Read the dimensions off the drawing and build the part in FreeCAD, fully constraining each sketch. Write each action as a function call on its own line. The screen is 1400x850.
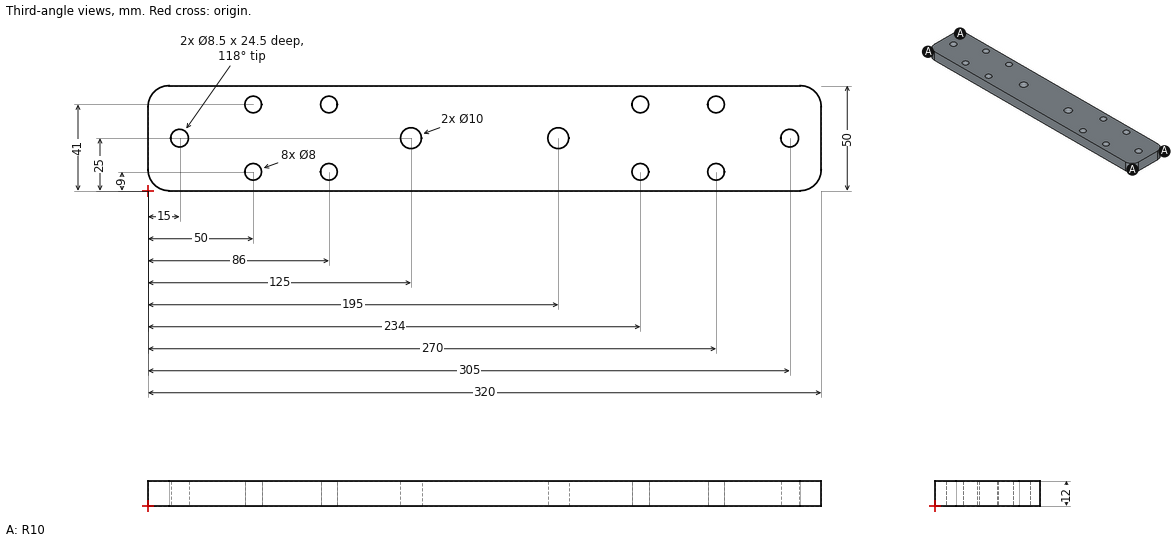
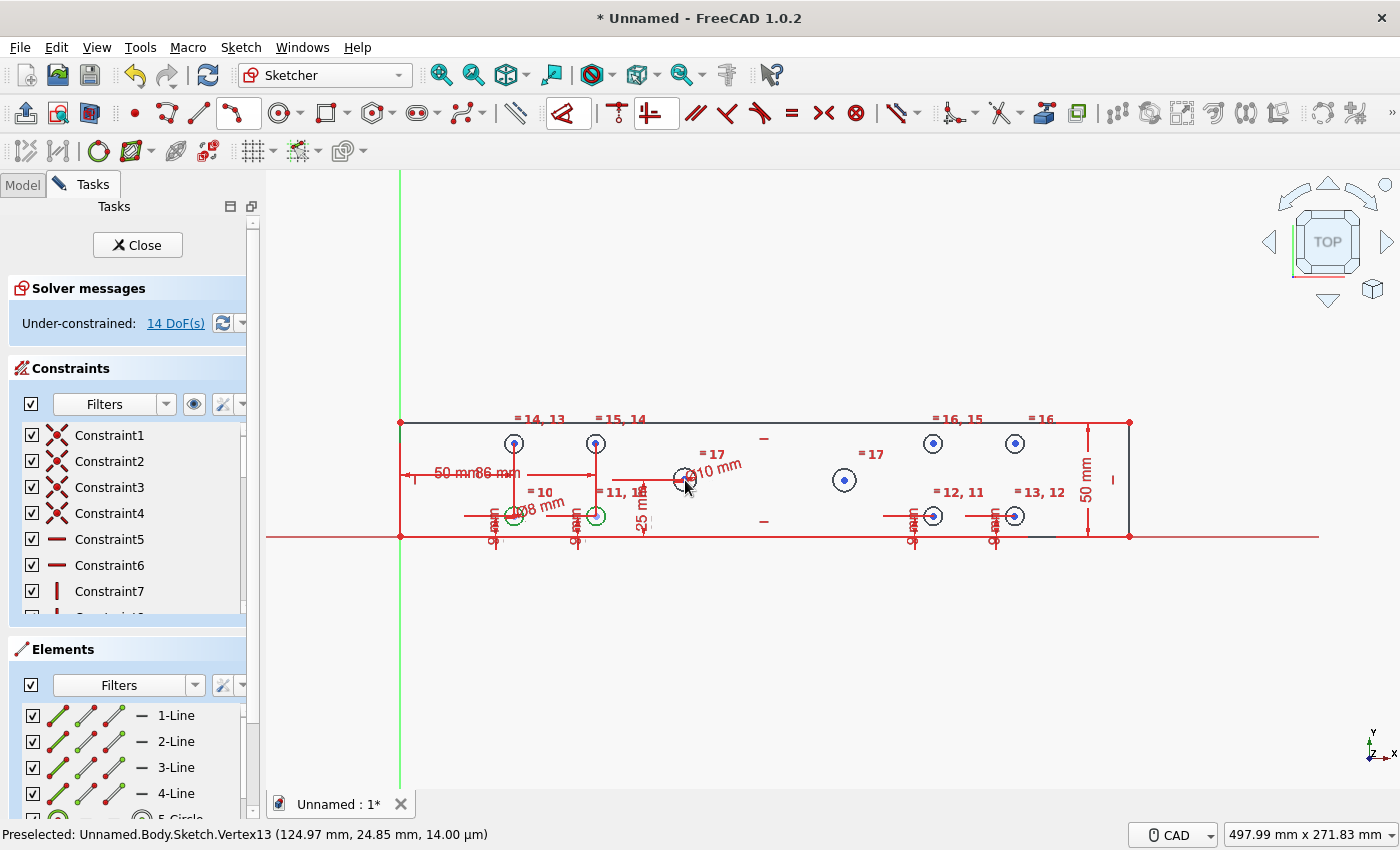
click(514, 444)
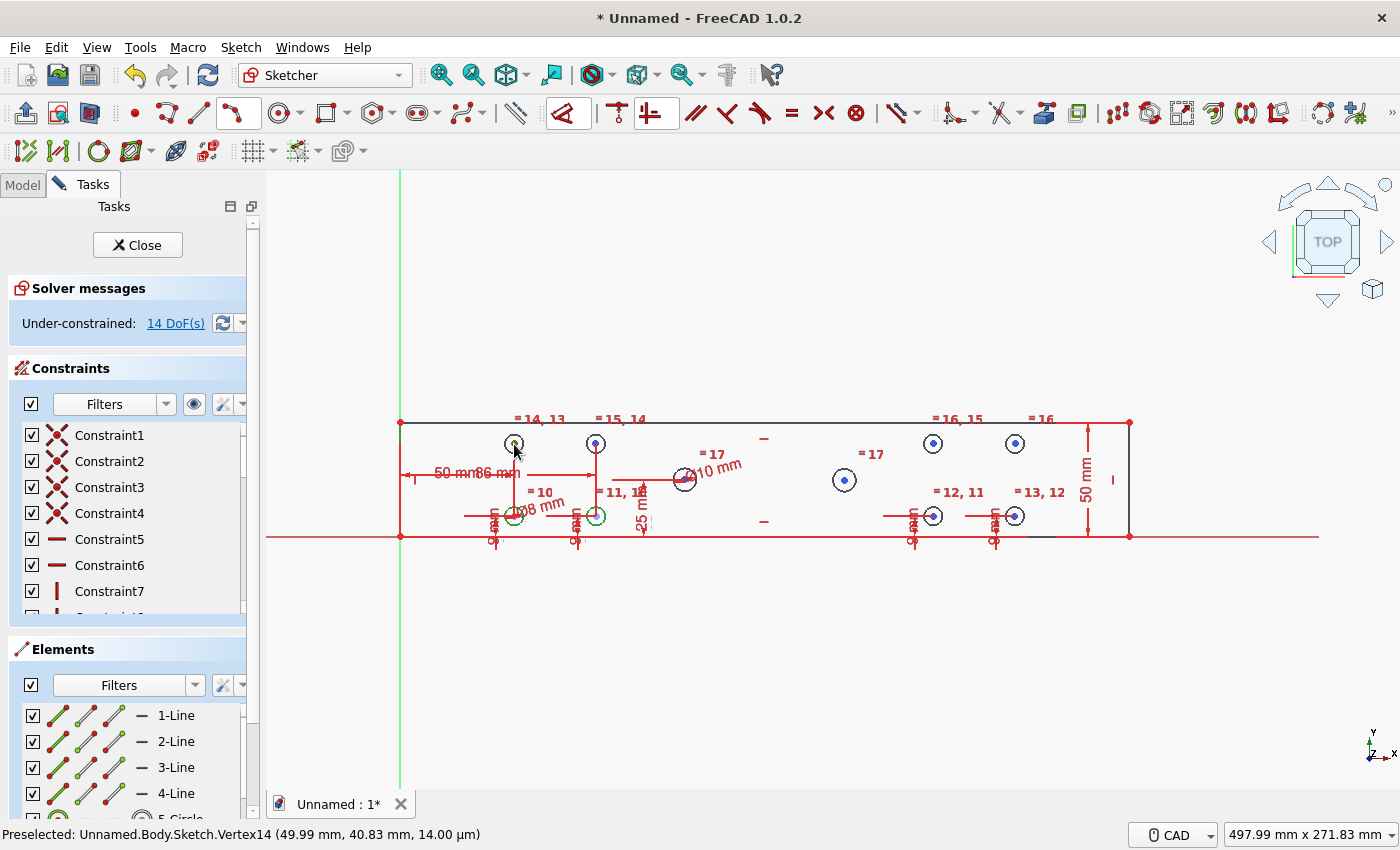
click(586, 114)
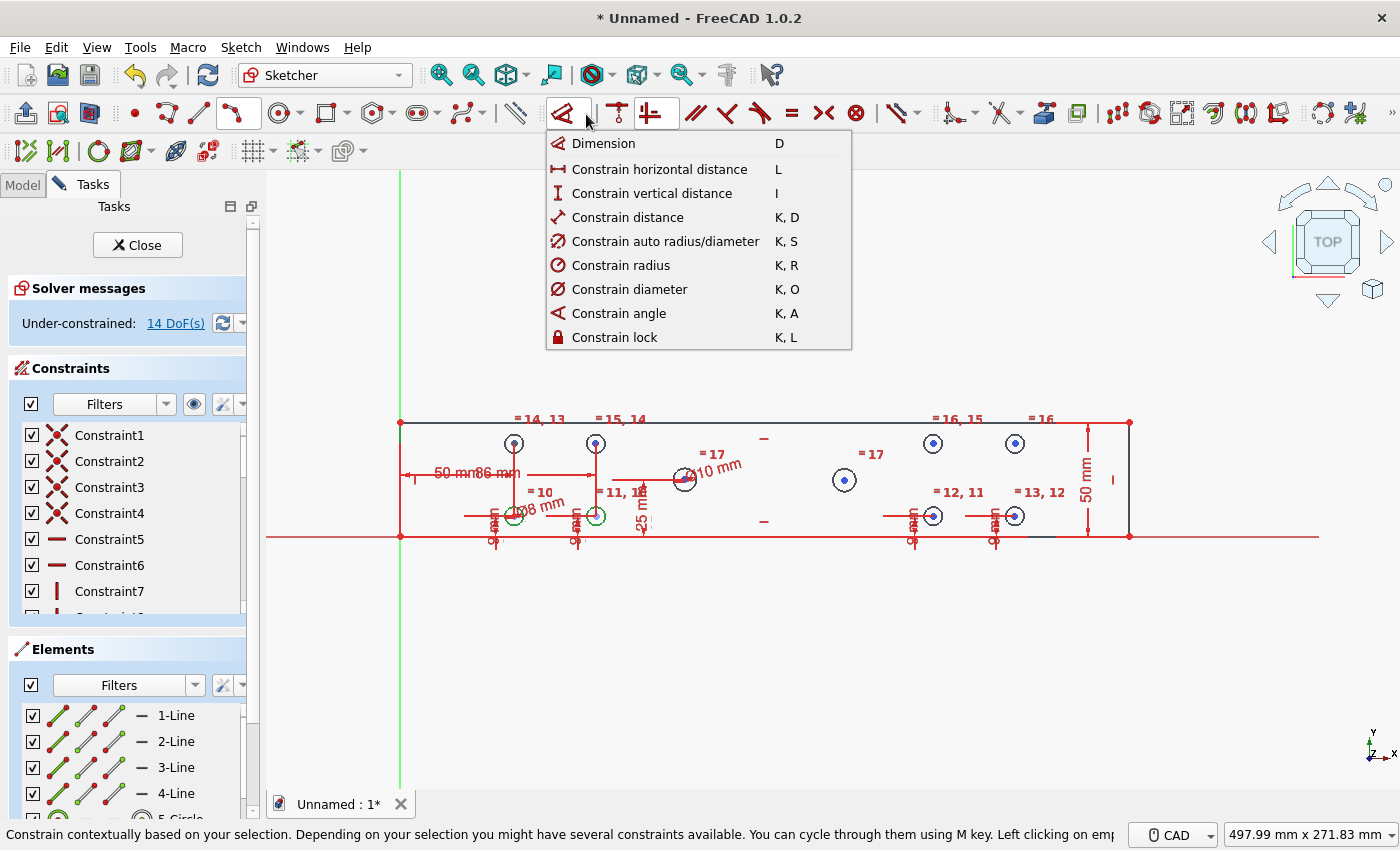
click(699, 169)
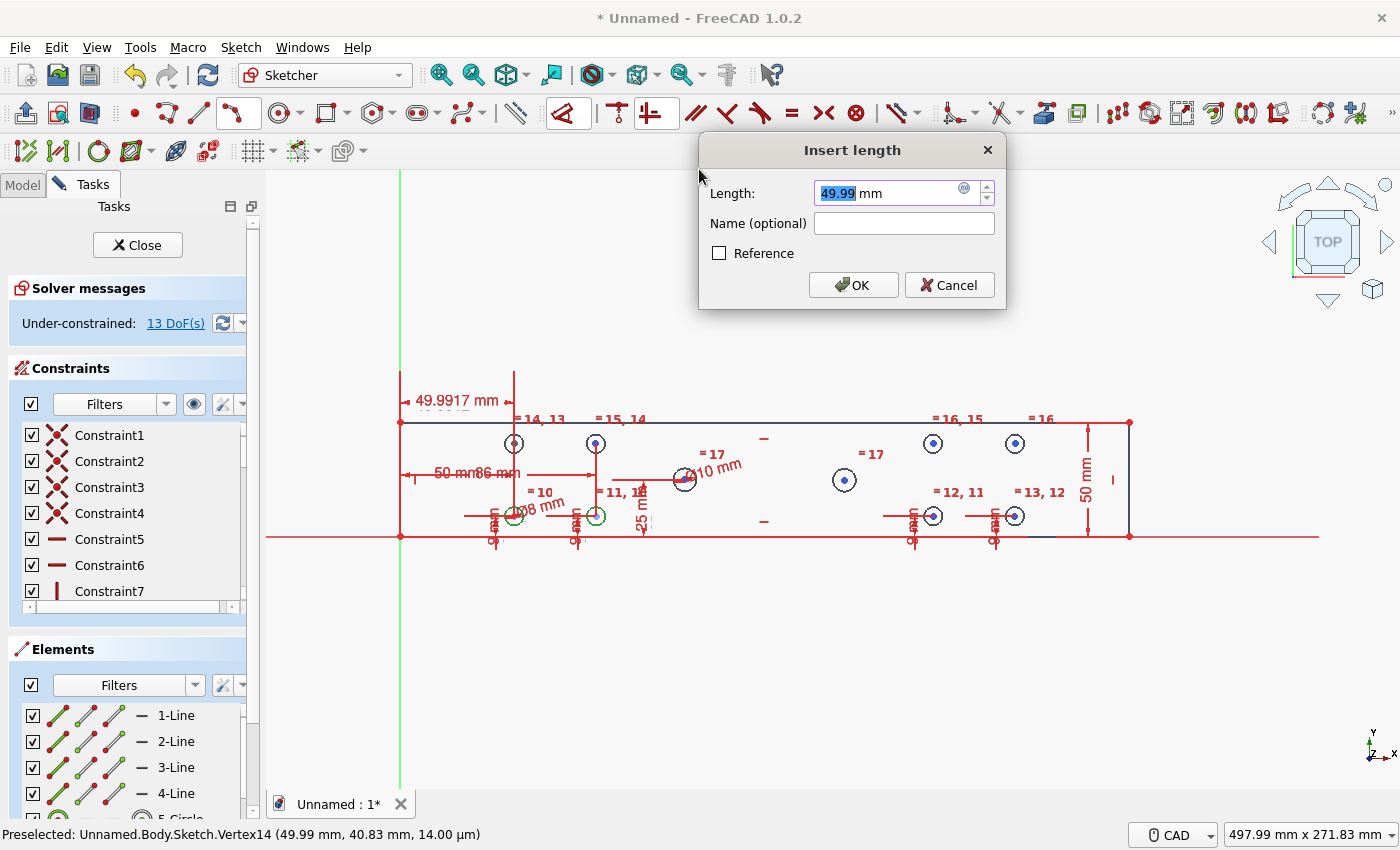
text(50)
key(Return)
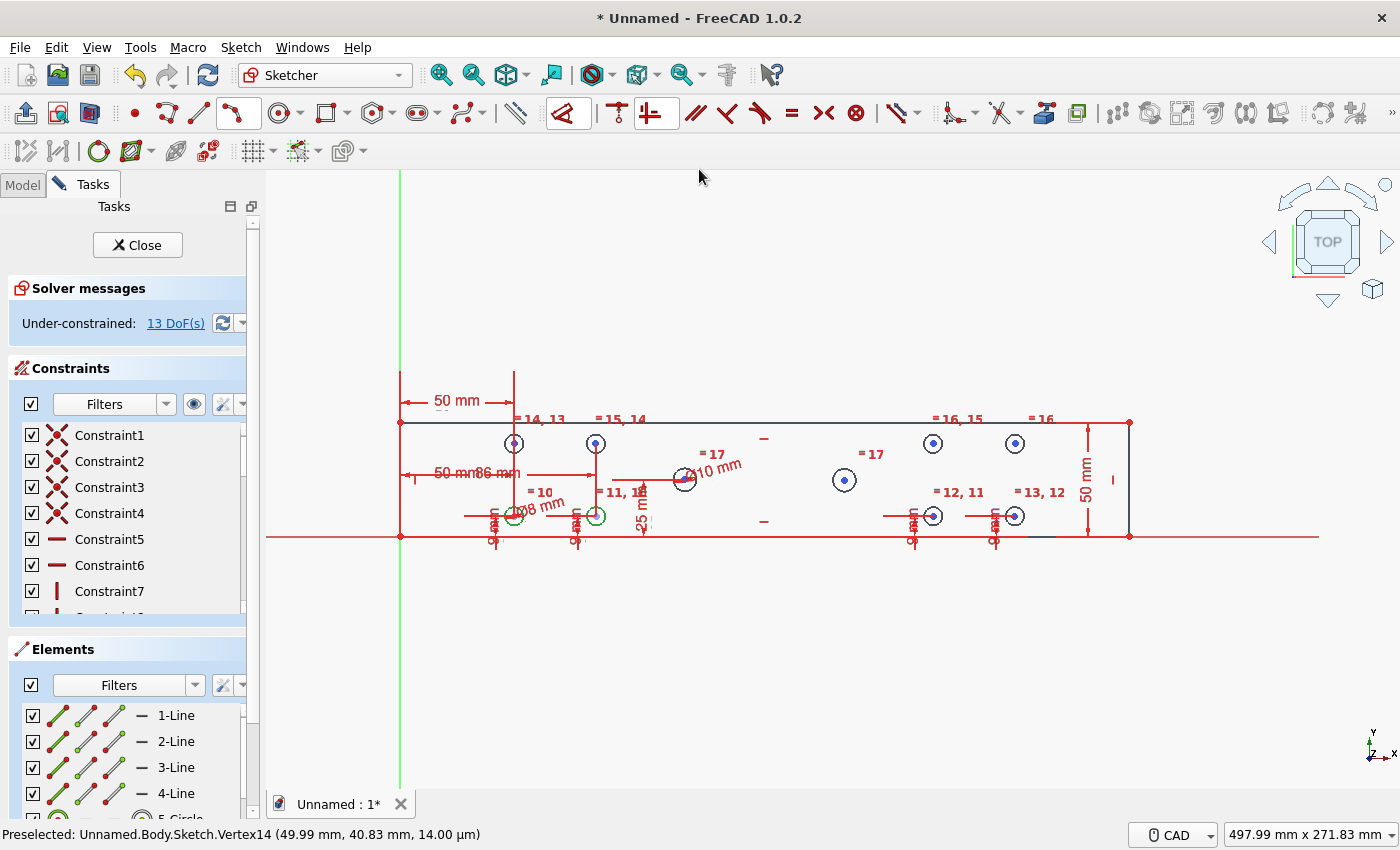
click(514, 444)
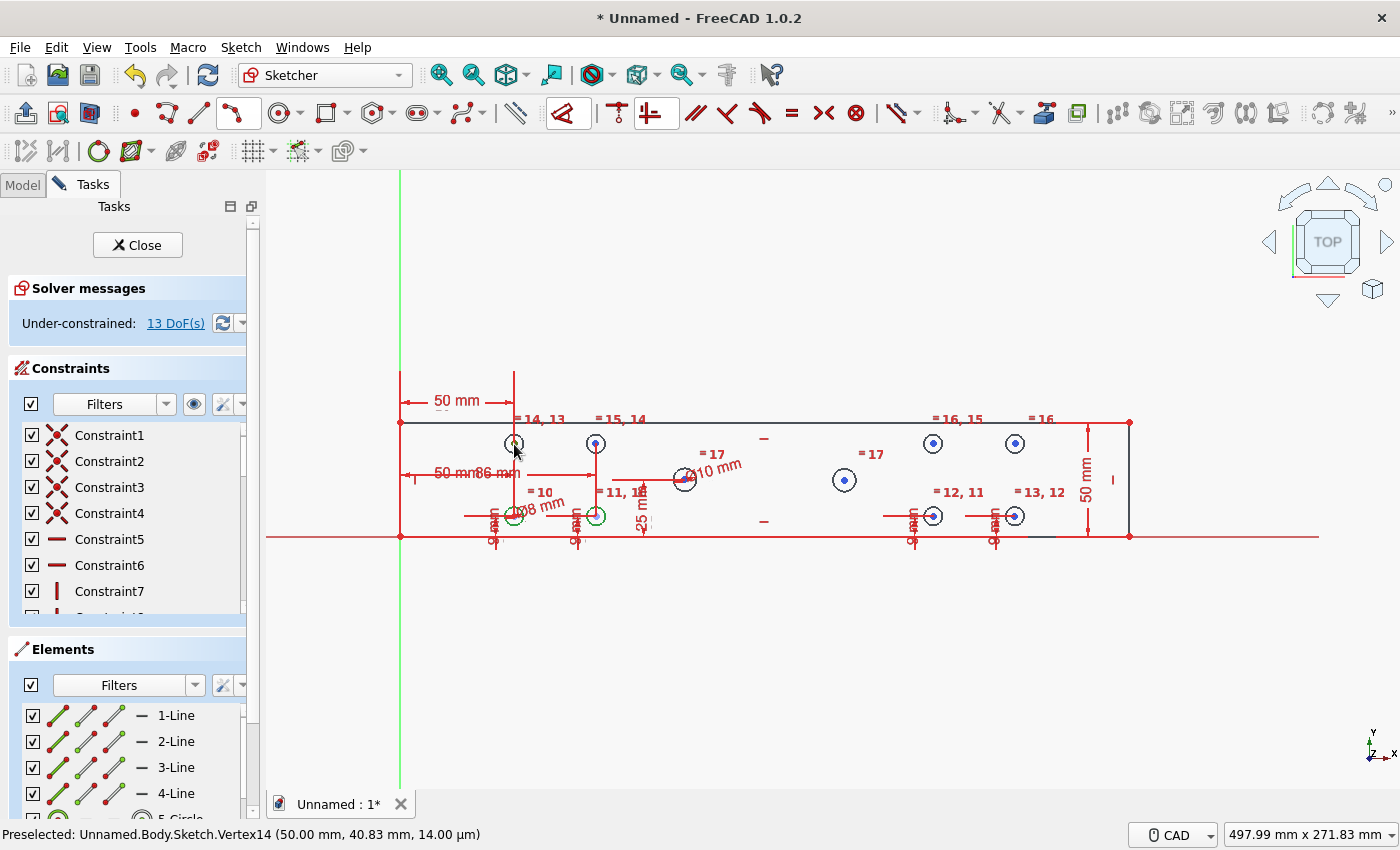
key(i)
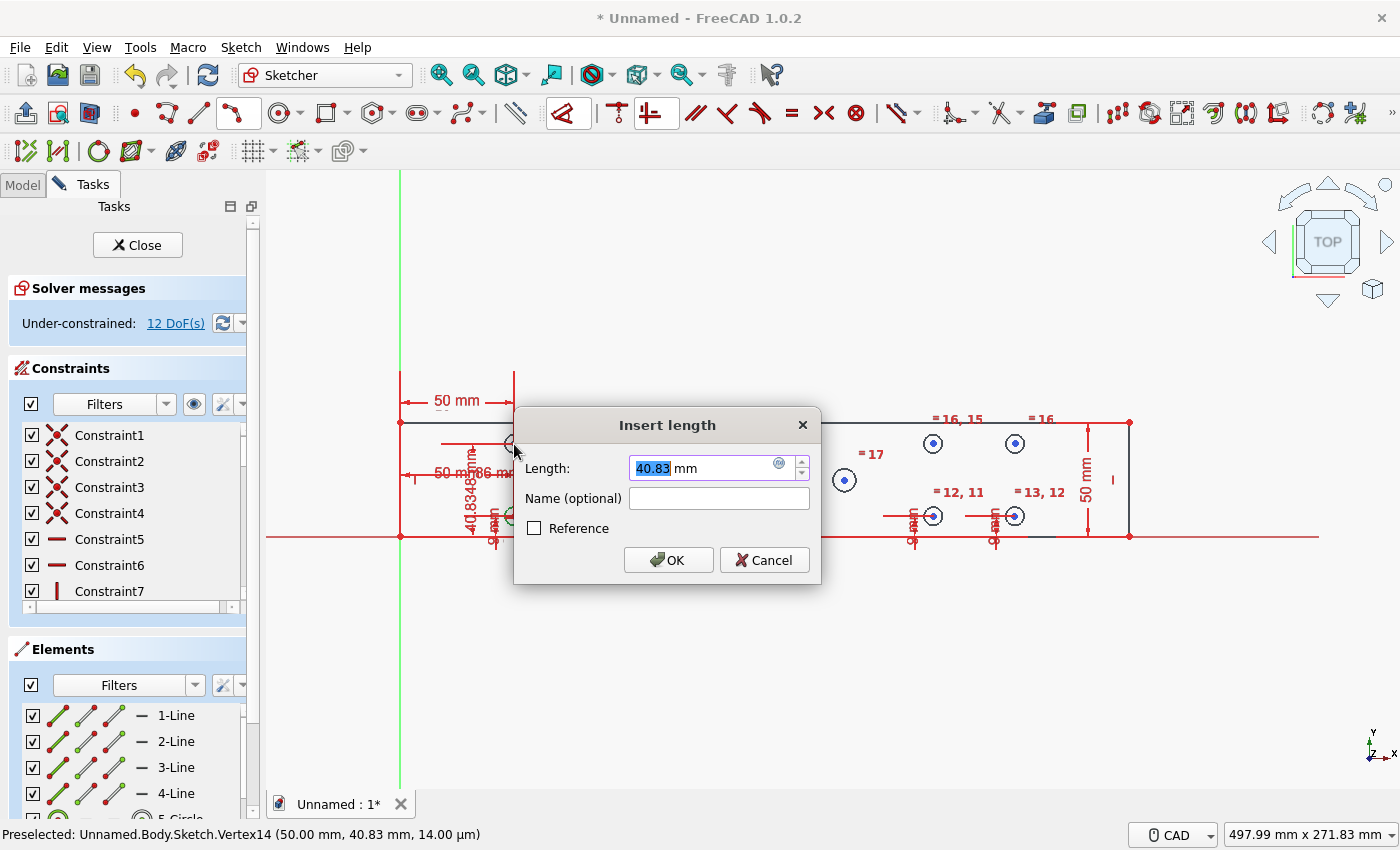
text(41)
key(Return)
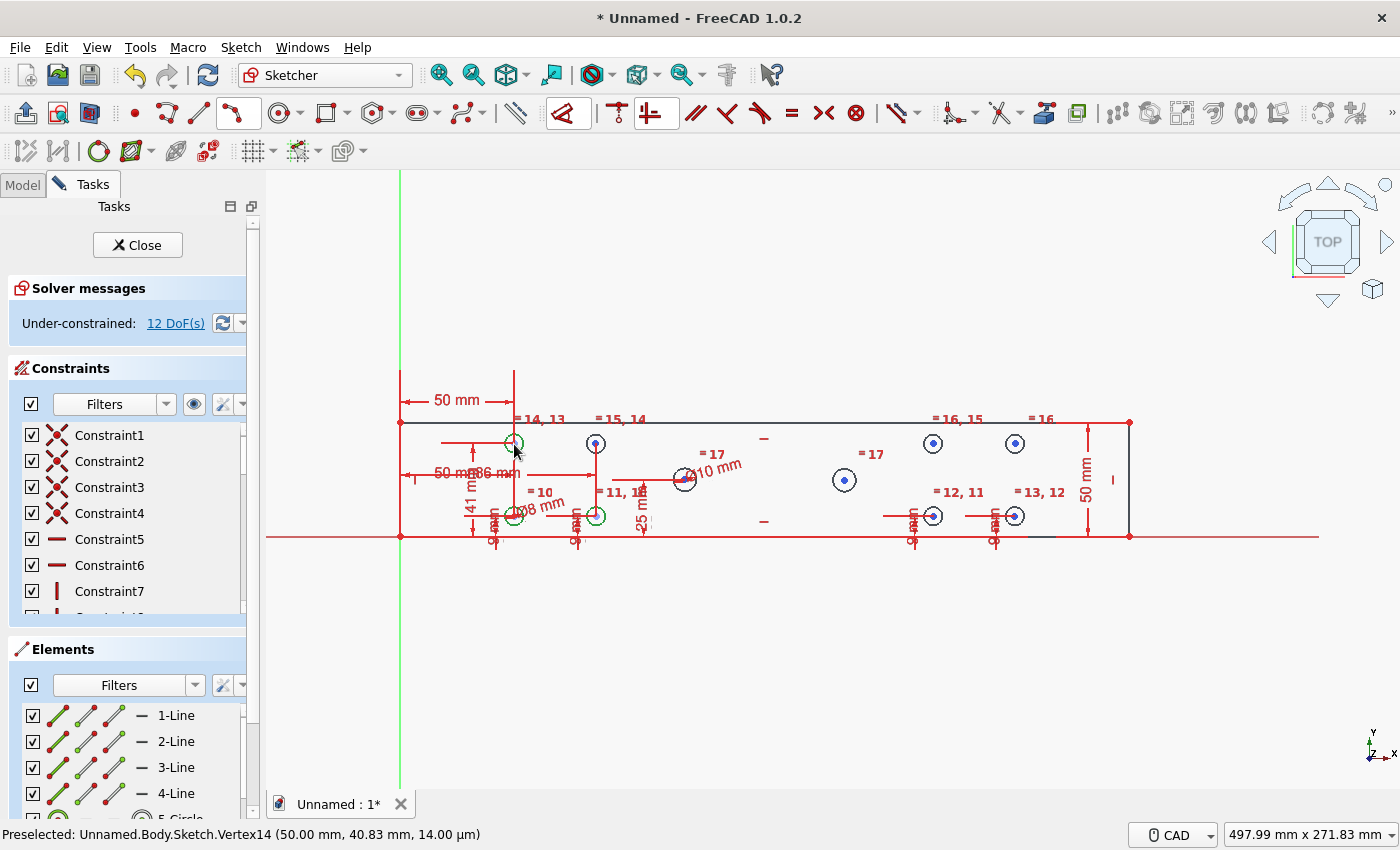
click(596, 444)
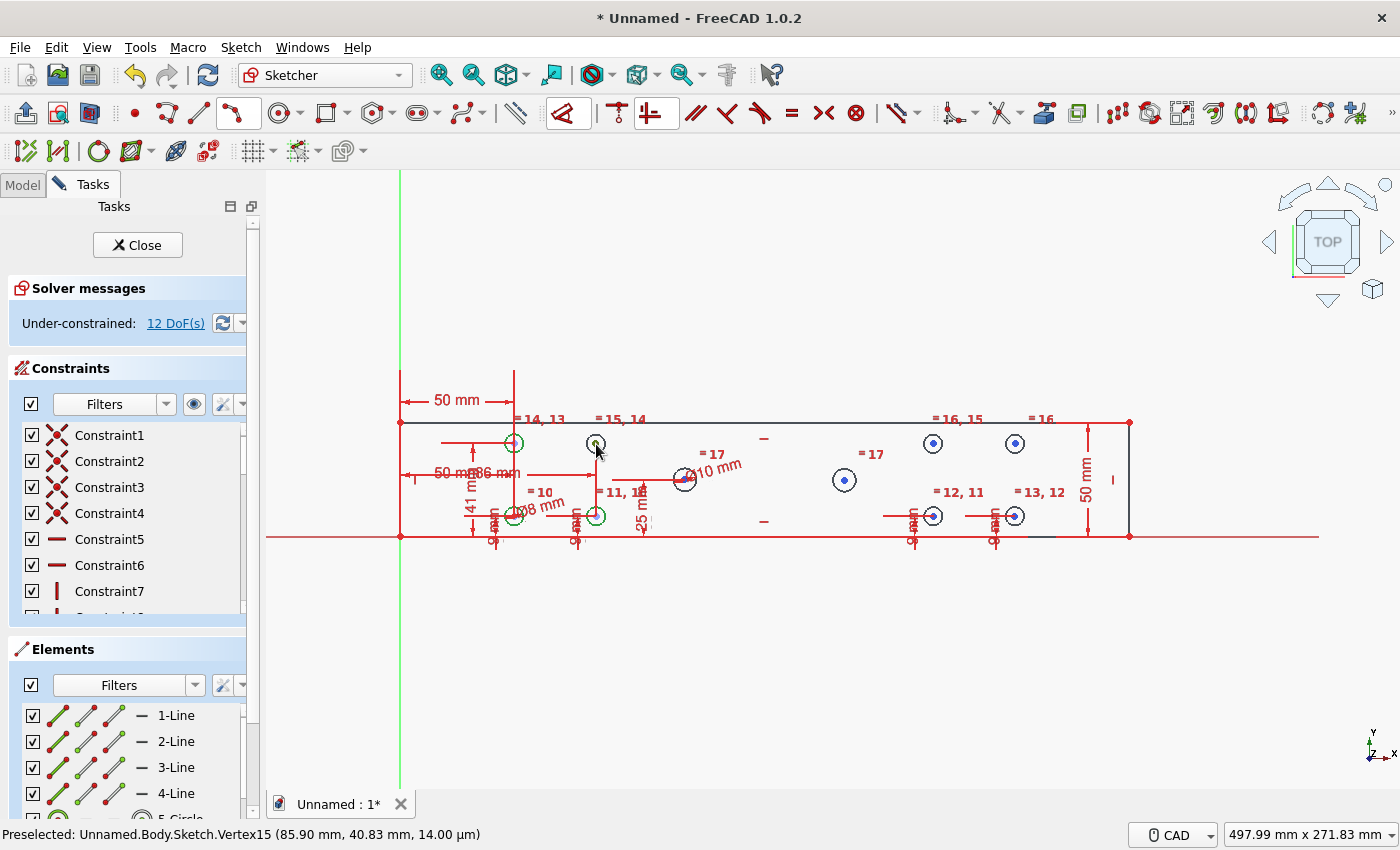
key(l)